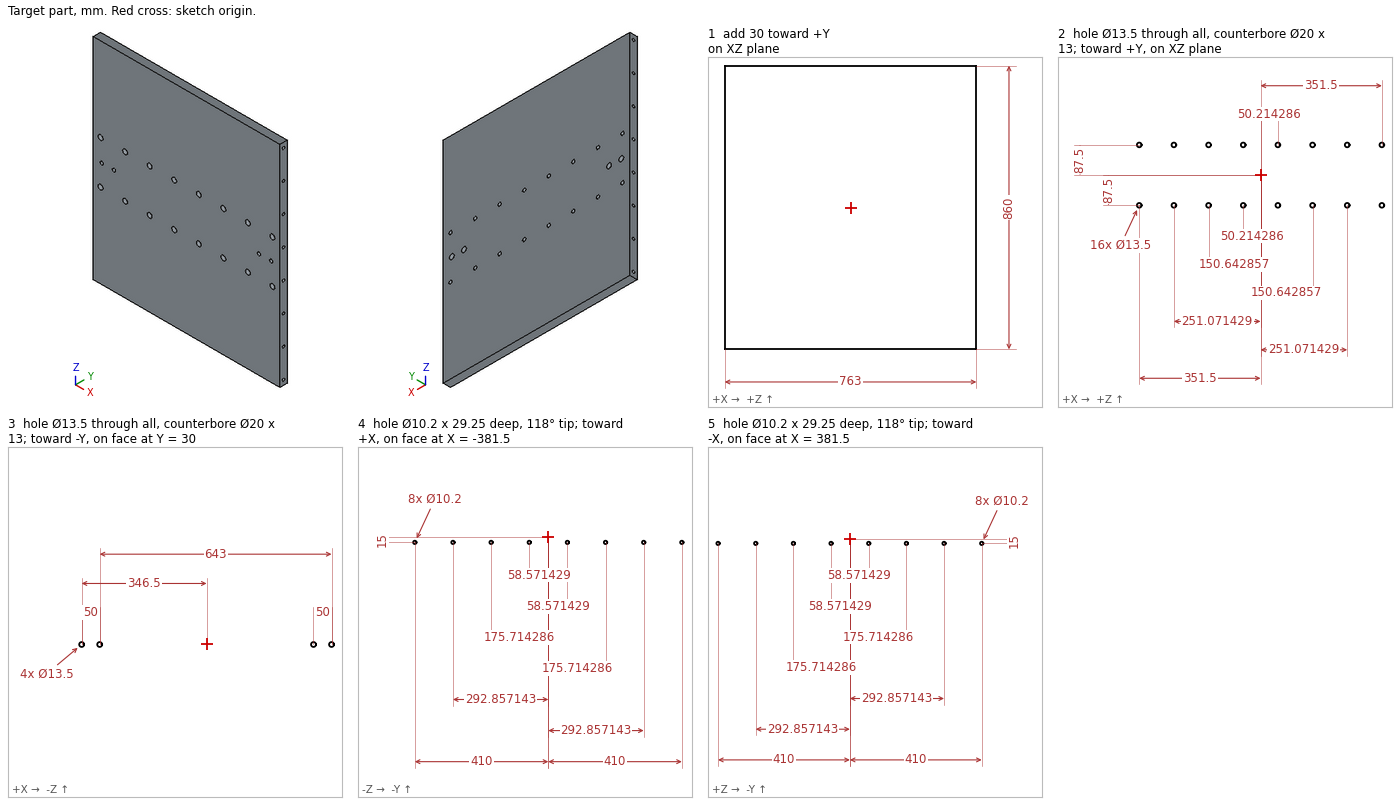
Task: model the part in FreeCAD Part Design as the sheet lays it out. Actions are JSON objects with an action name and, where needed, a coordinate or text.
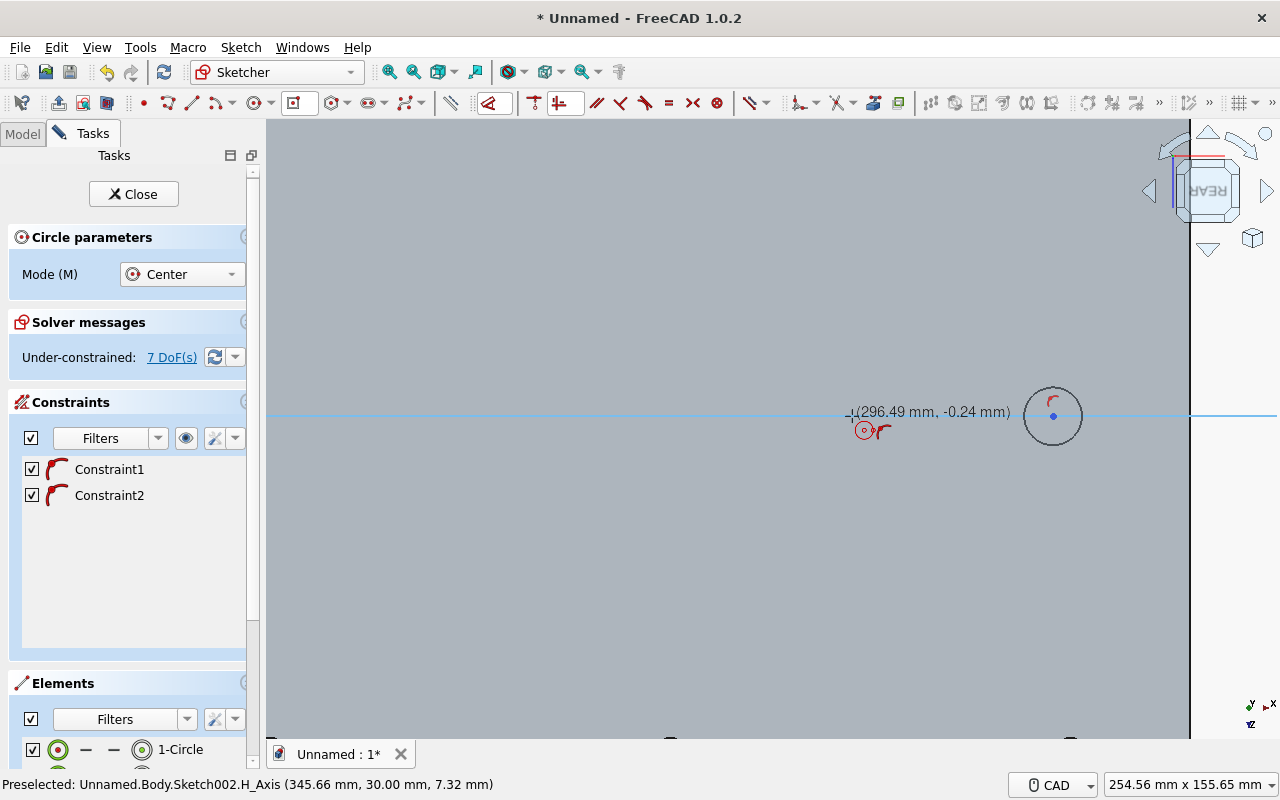
{"action": "scroll", "coordinate": [966, 432], "scroll_direction": "down", "scroll_amount": 8}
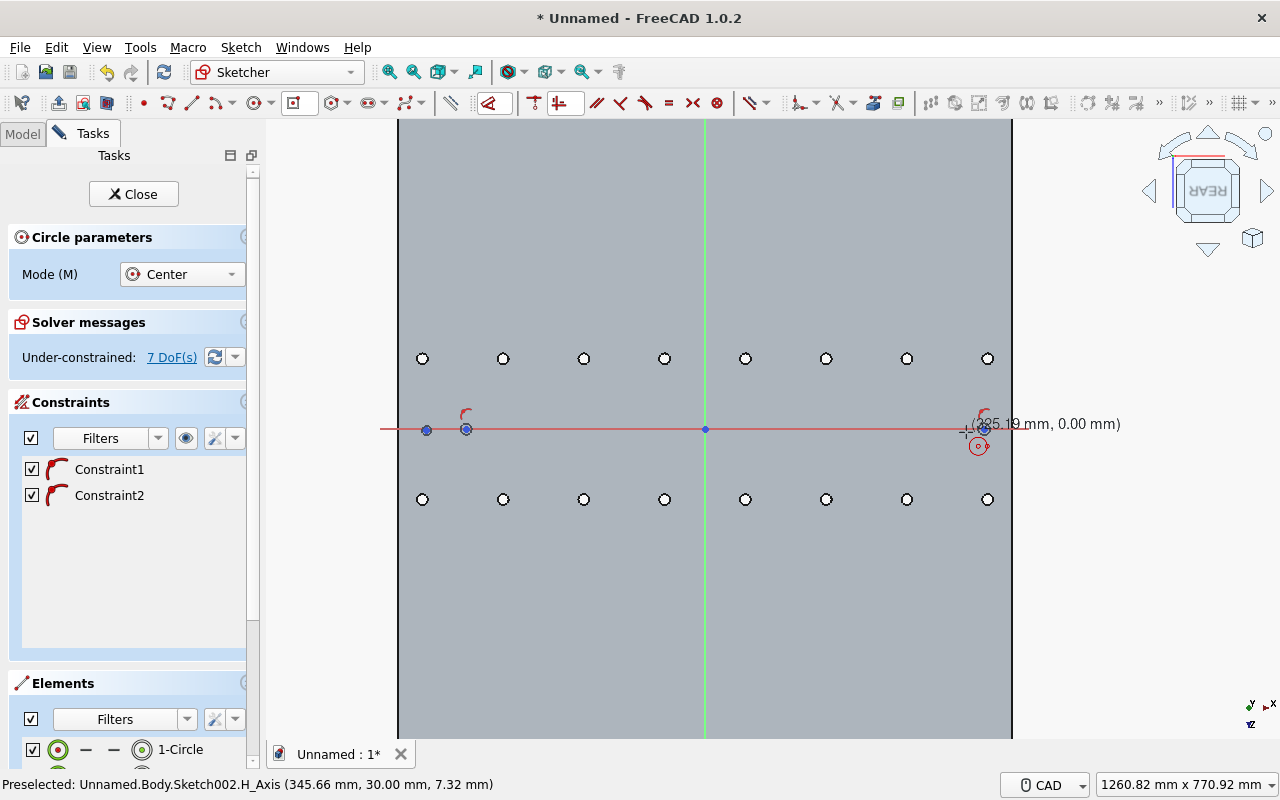
{"action": "left_click", "coordinate": [943, 429]}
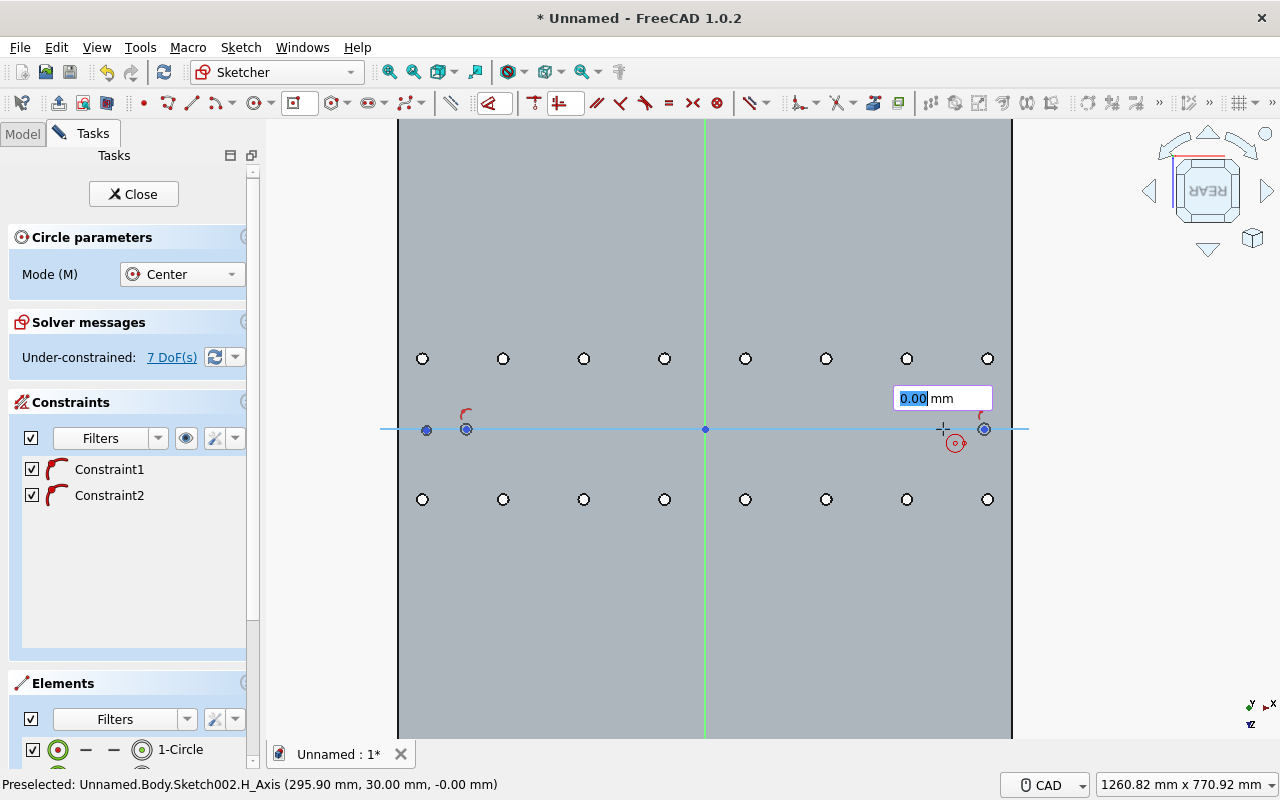
{"action": "scroll", "coordinate": [942, 434], "scroll_direction": "up", "scroll_amount": 6}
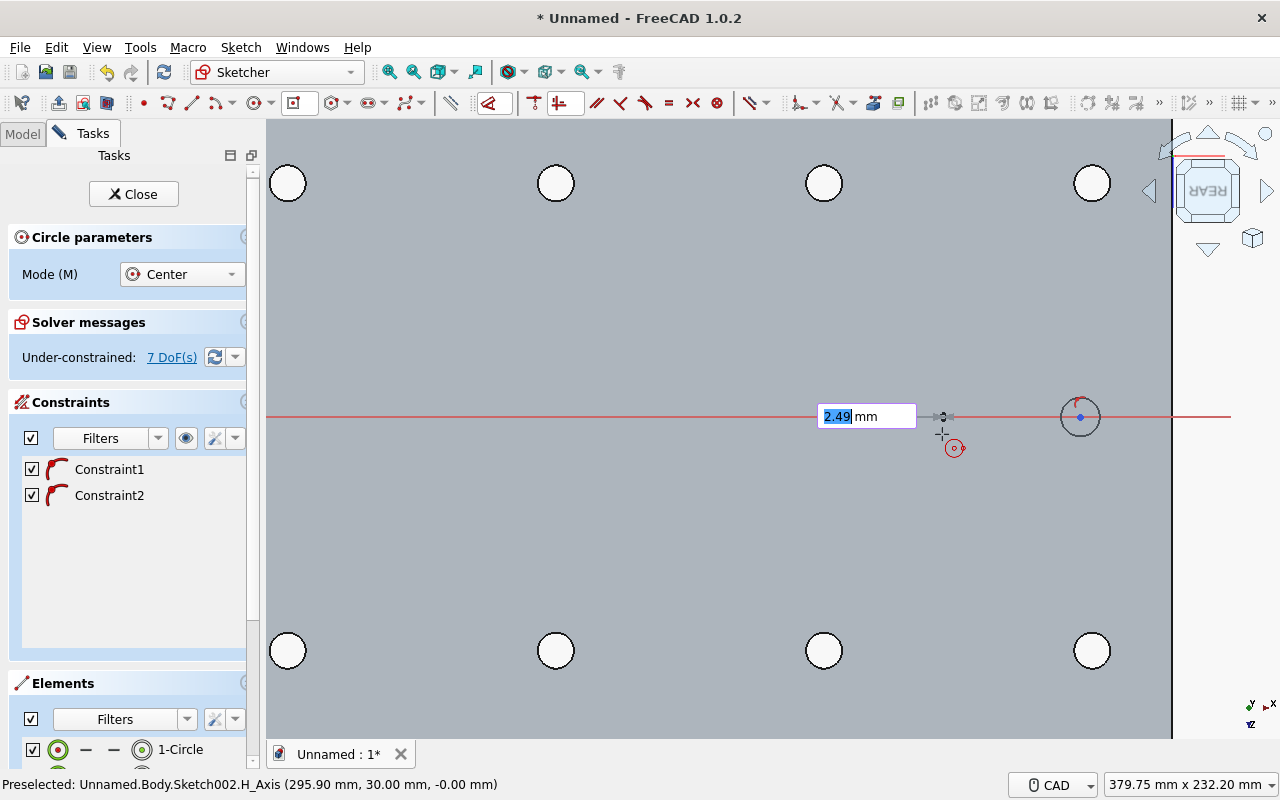
{"action": "left_click", "coordinate": [939, 434]}
{"action": "key", "text": "Escape"}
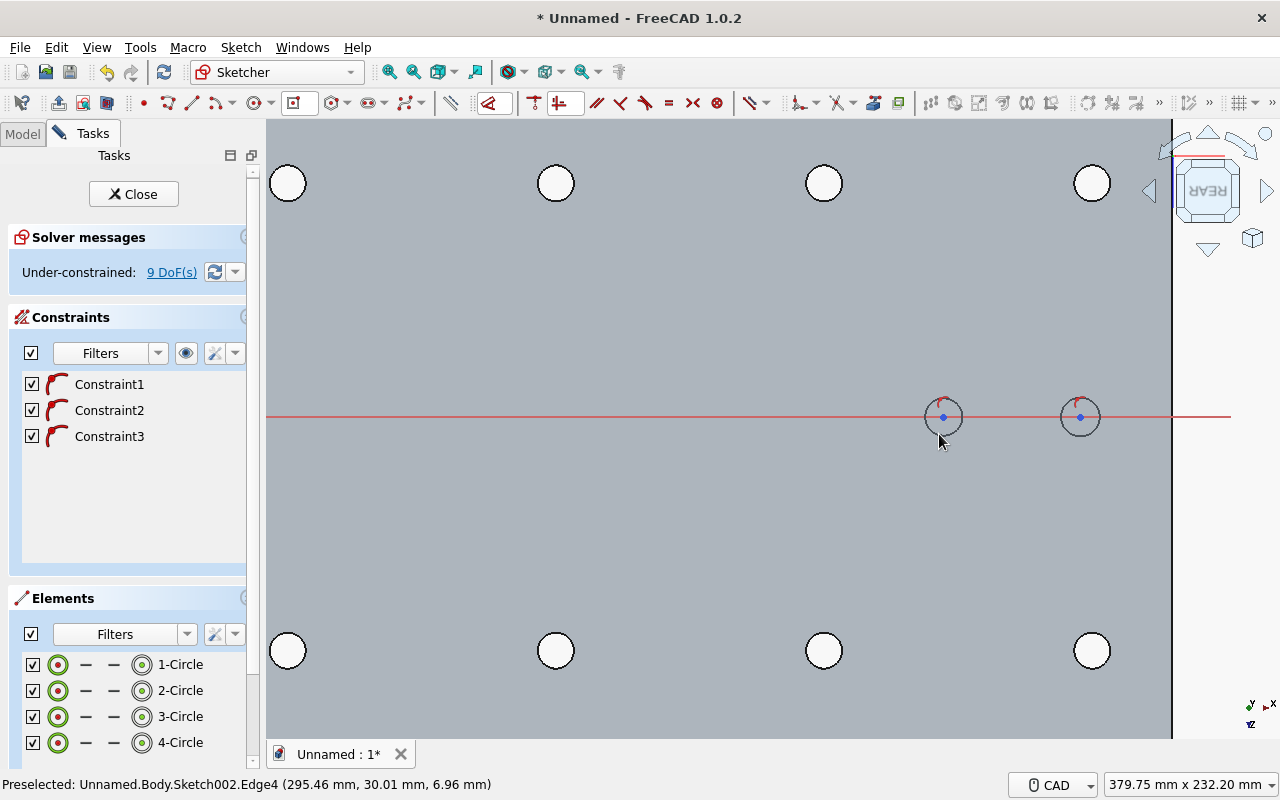
{"action": "scroll", "coordinate": [942, 434], "scroll_direction": "down", "scroll_amount": 6}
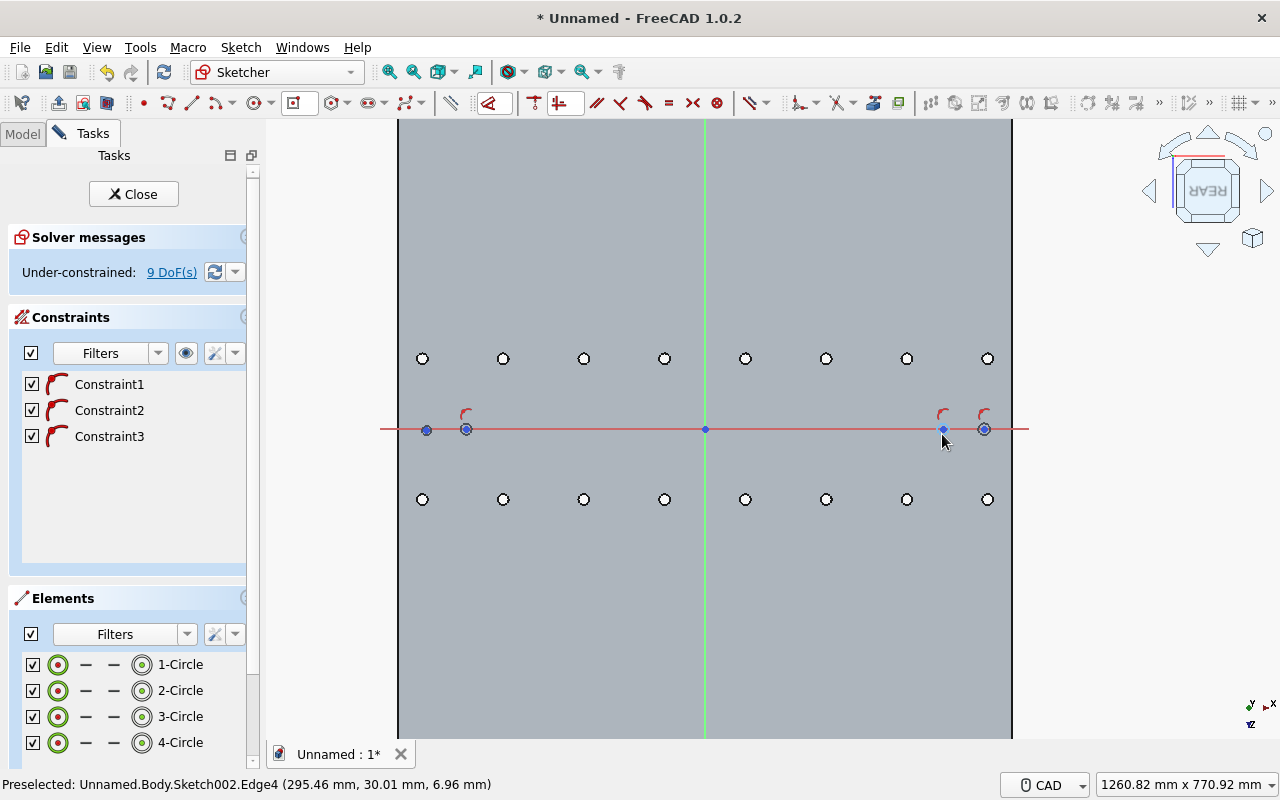
{"action": "scroll", "coordinate": [423, 434], "scroll_direction": "up", "scroll_amount": 6}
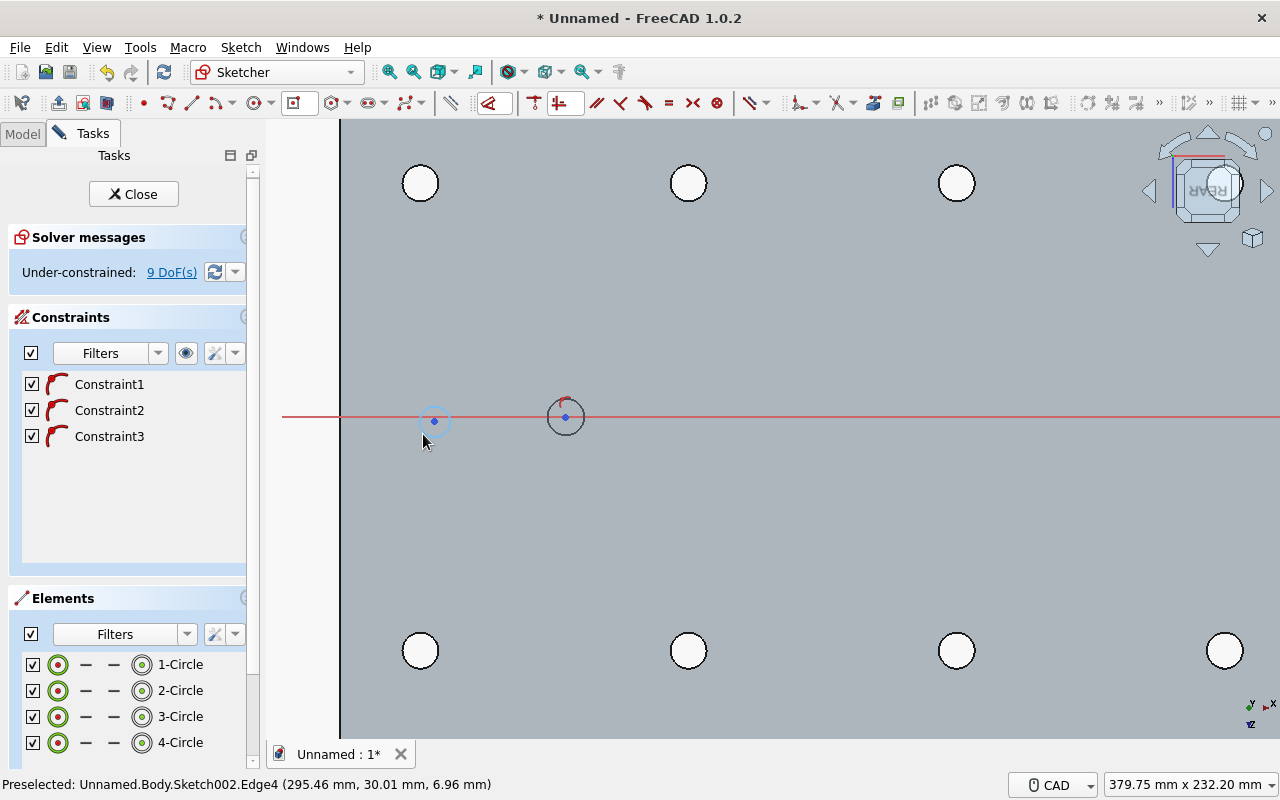
{"action": "left_click", "coordinate": [424, 433]}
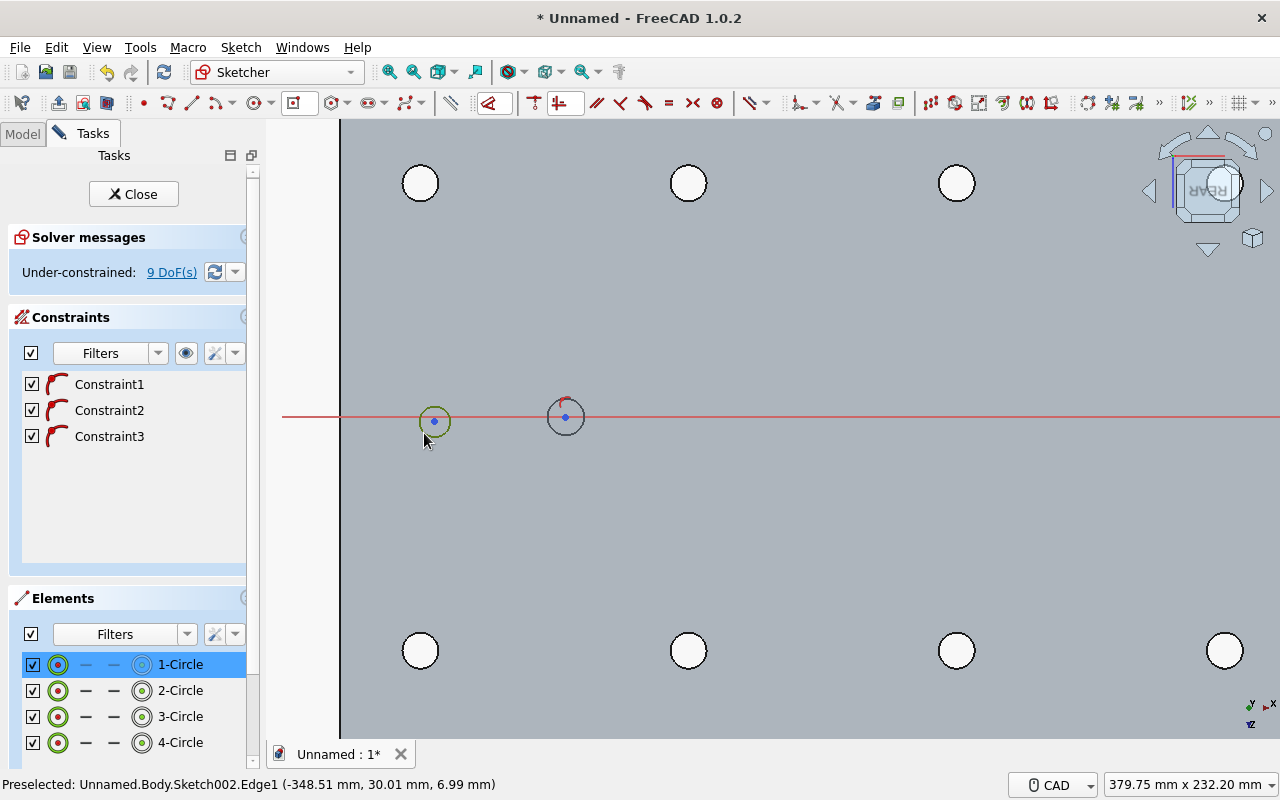
{"action": "left_click", "coordinate": [579, 404]}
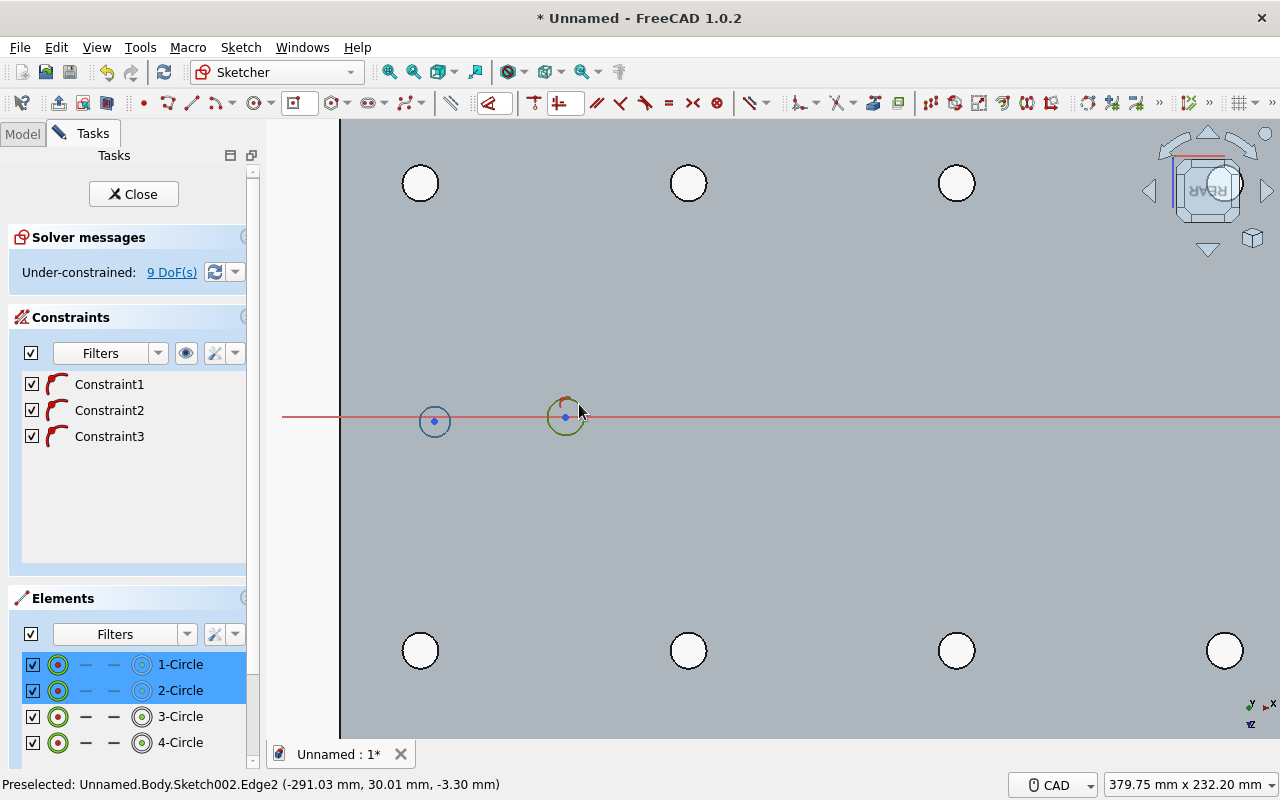
{"action": "scroll", "coordinate": [422, 434], "scroll_direction": "down", "scroll_amount": 6}